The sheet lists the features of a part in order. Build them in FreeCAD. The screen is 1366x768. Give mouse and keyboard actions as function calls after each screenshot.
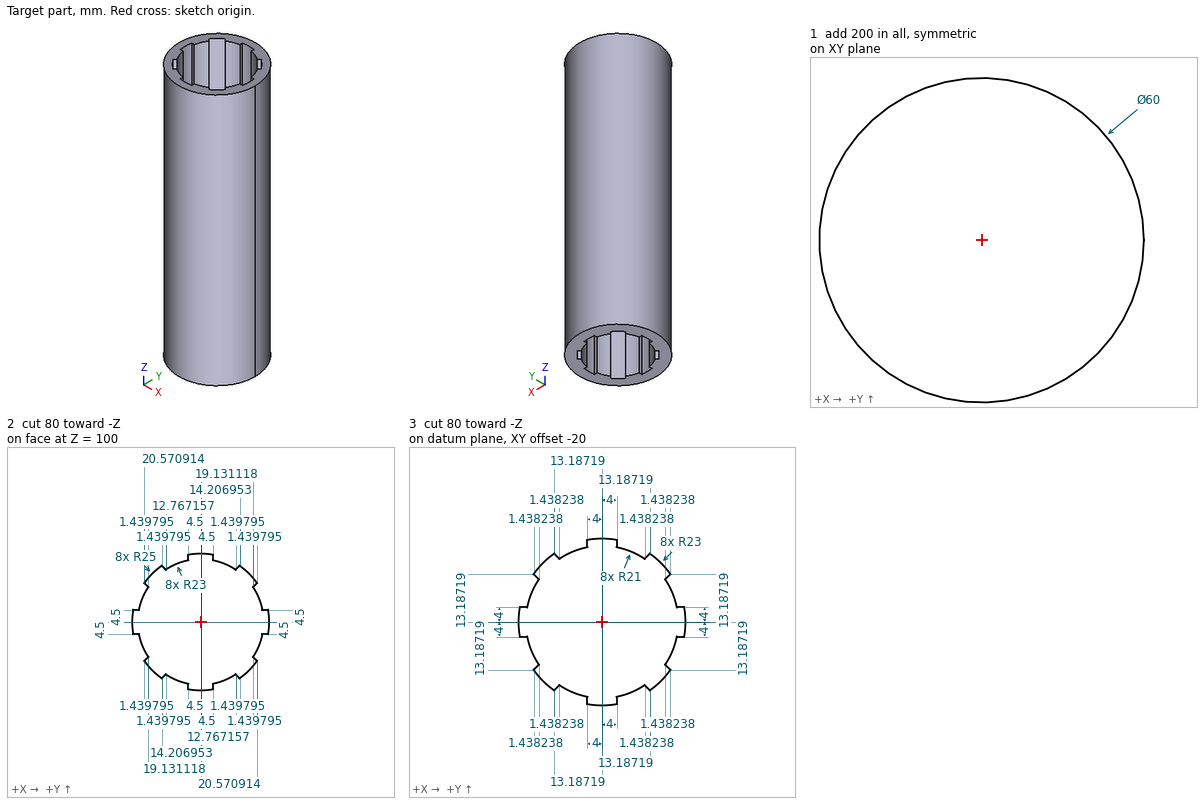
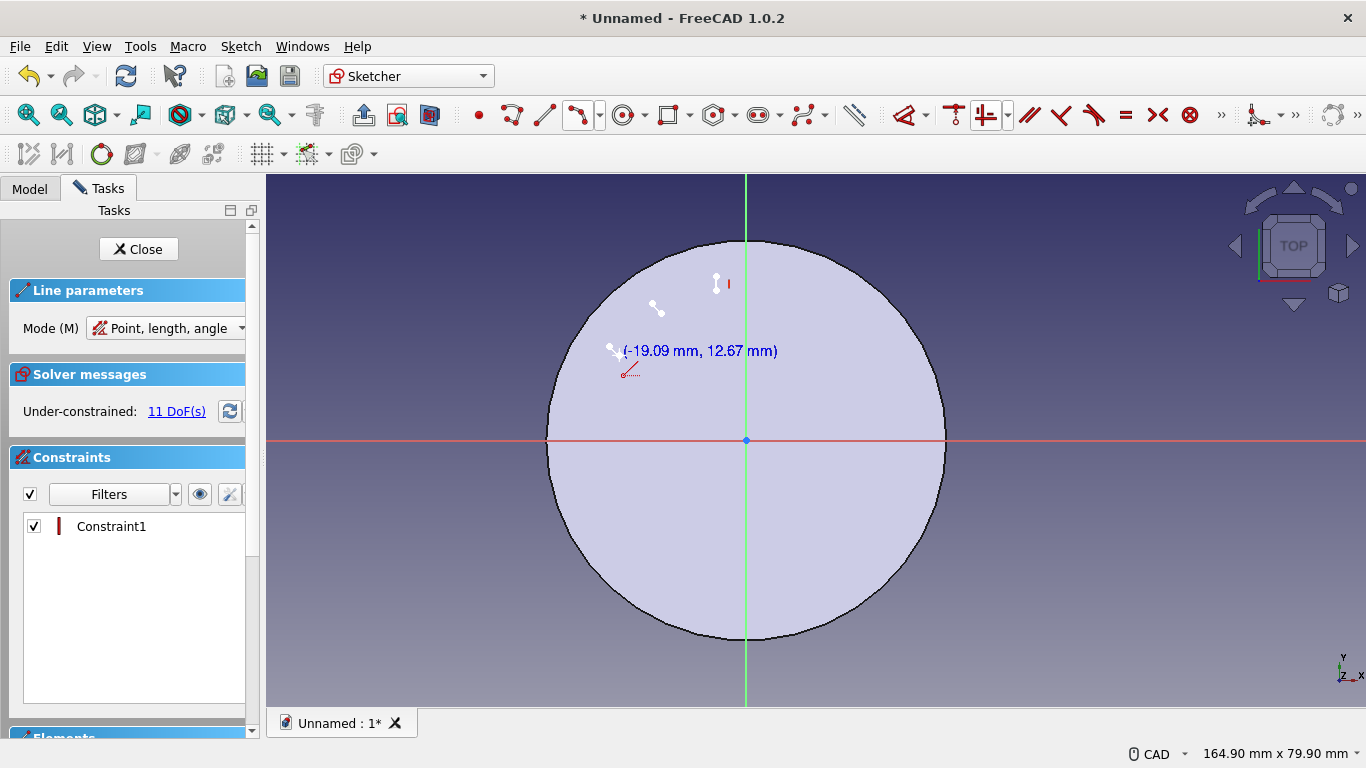
click(596, 410)
click(582, 410)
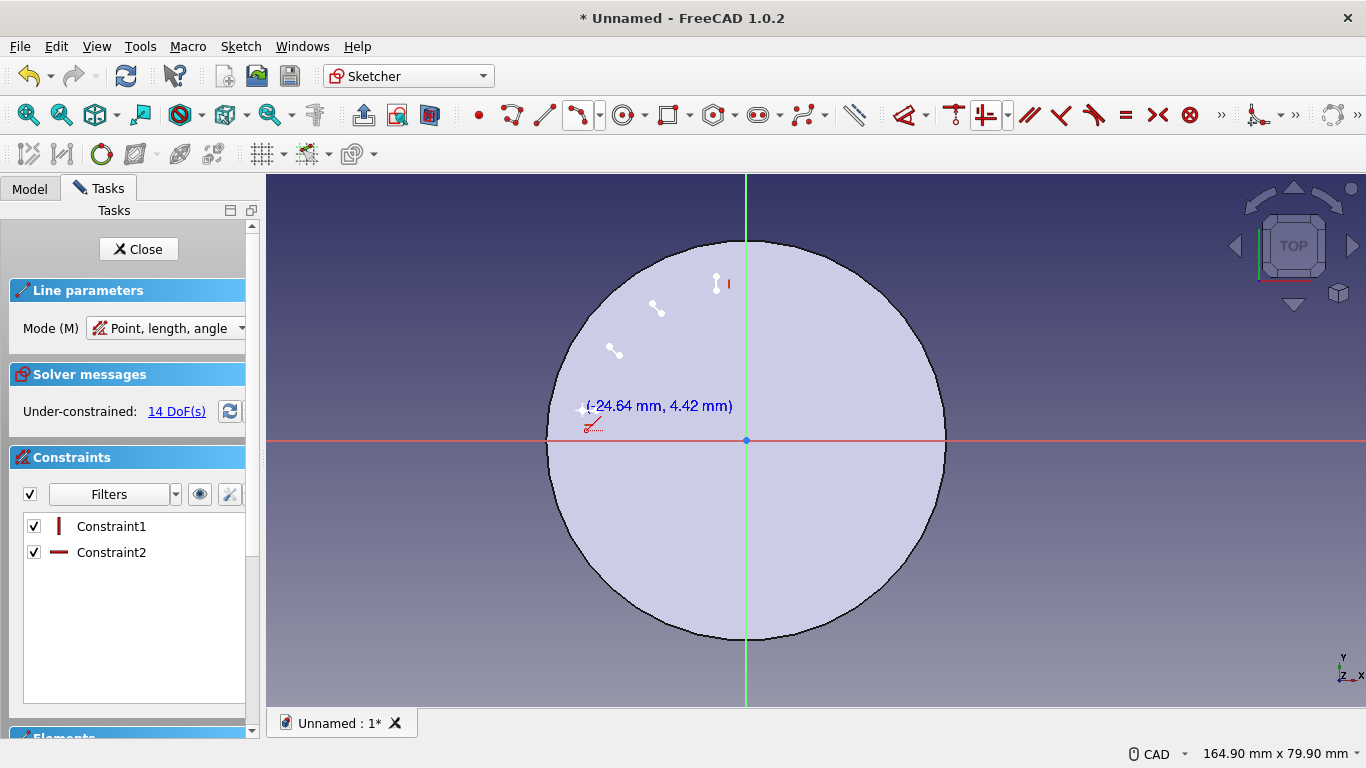
click(582, 471)
click(596, 471)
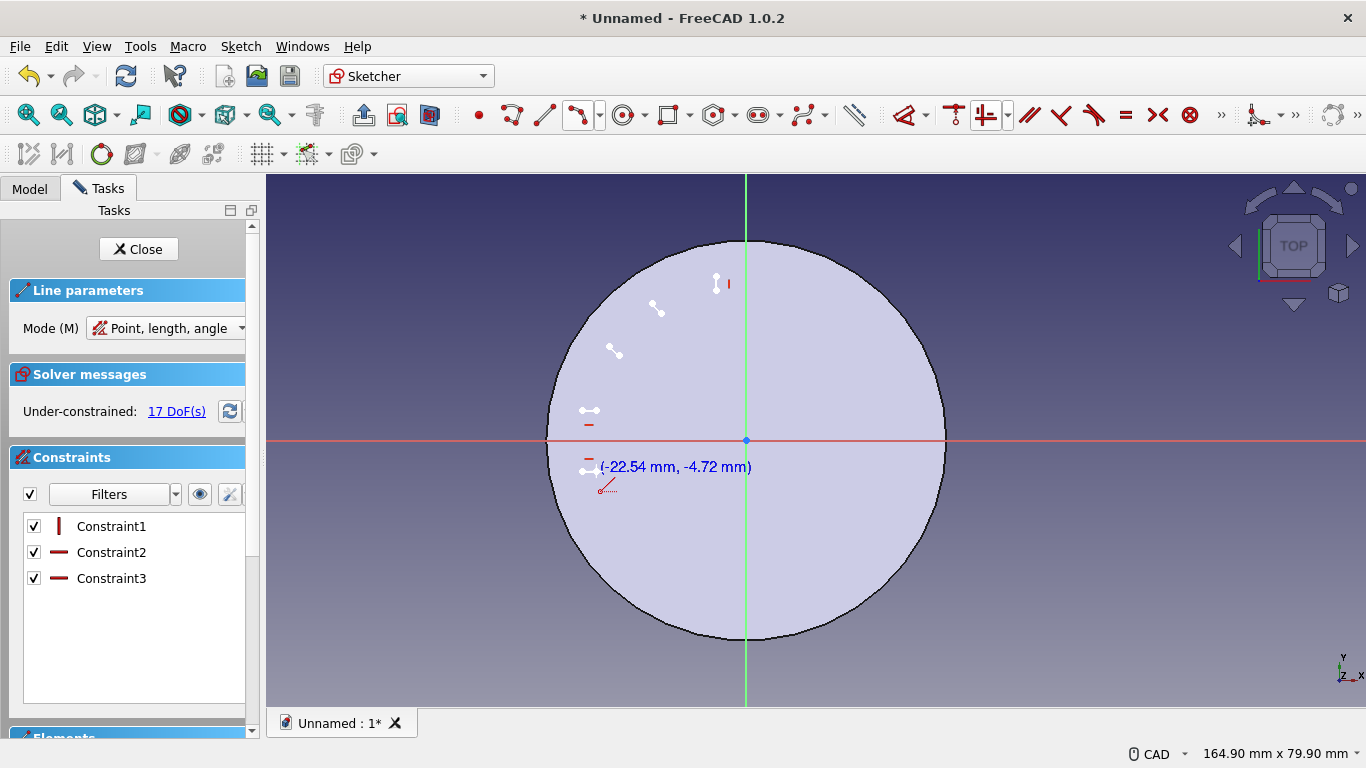
click(619, 526)
click(609, 535)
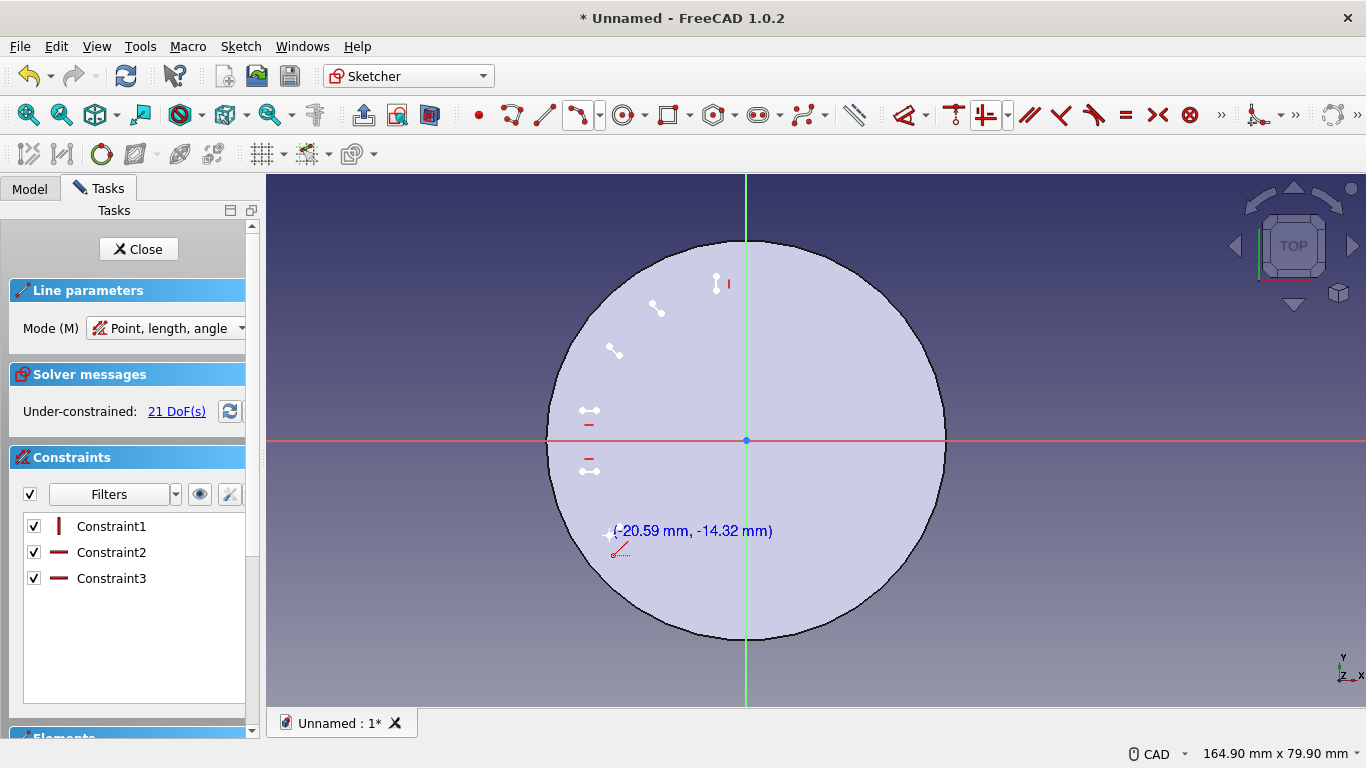
click(652, 578)
click(661, 568)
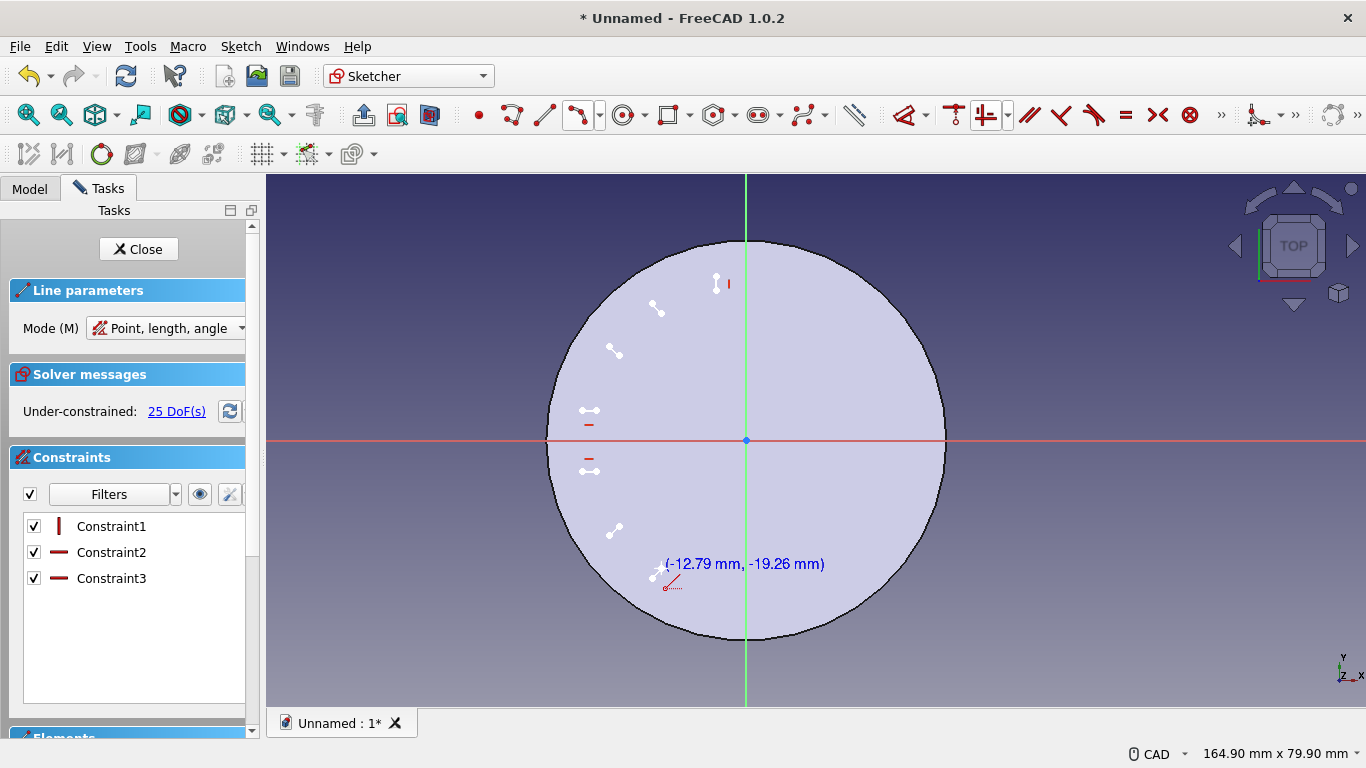
click(716, 591)
click(716, 605)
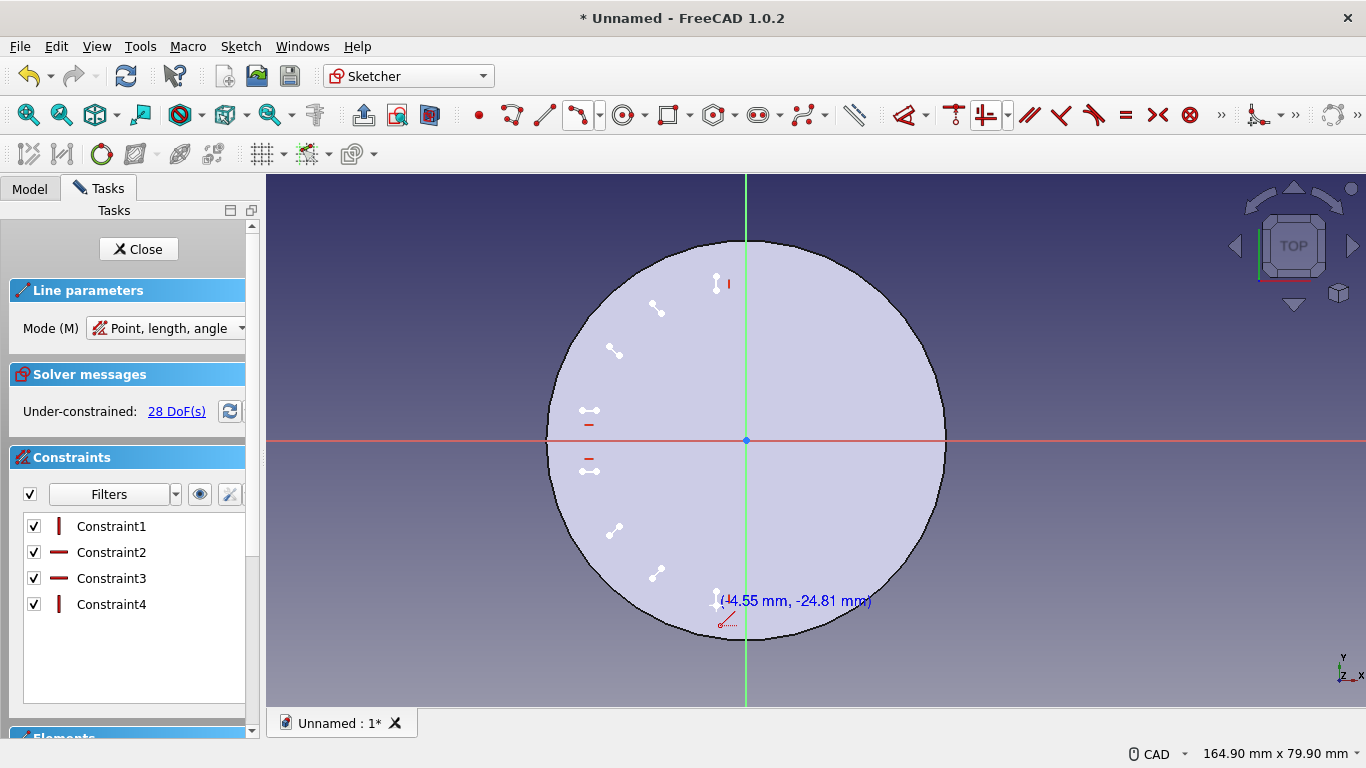
click(776, 605)
click(776, 591)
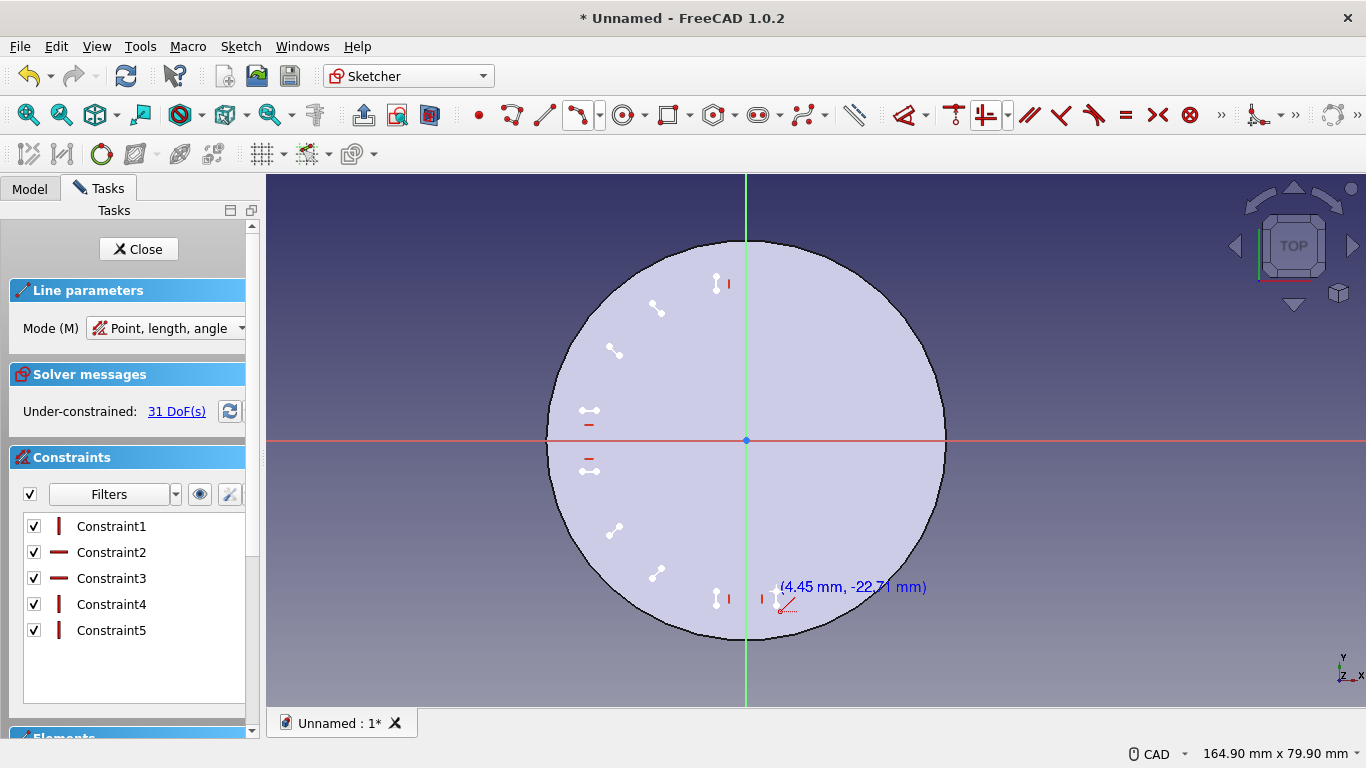
click(832, 568)
click(841, 578)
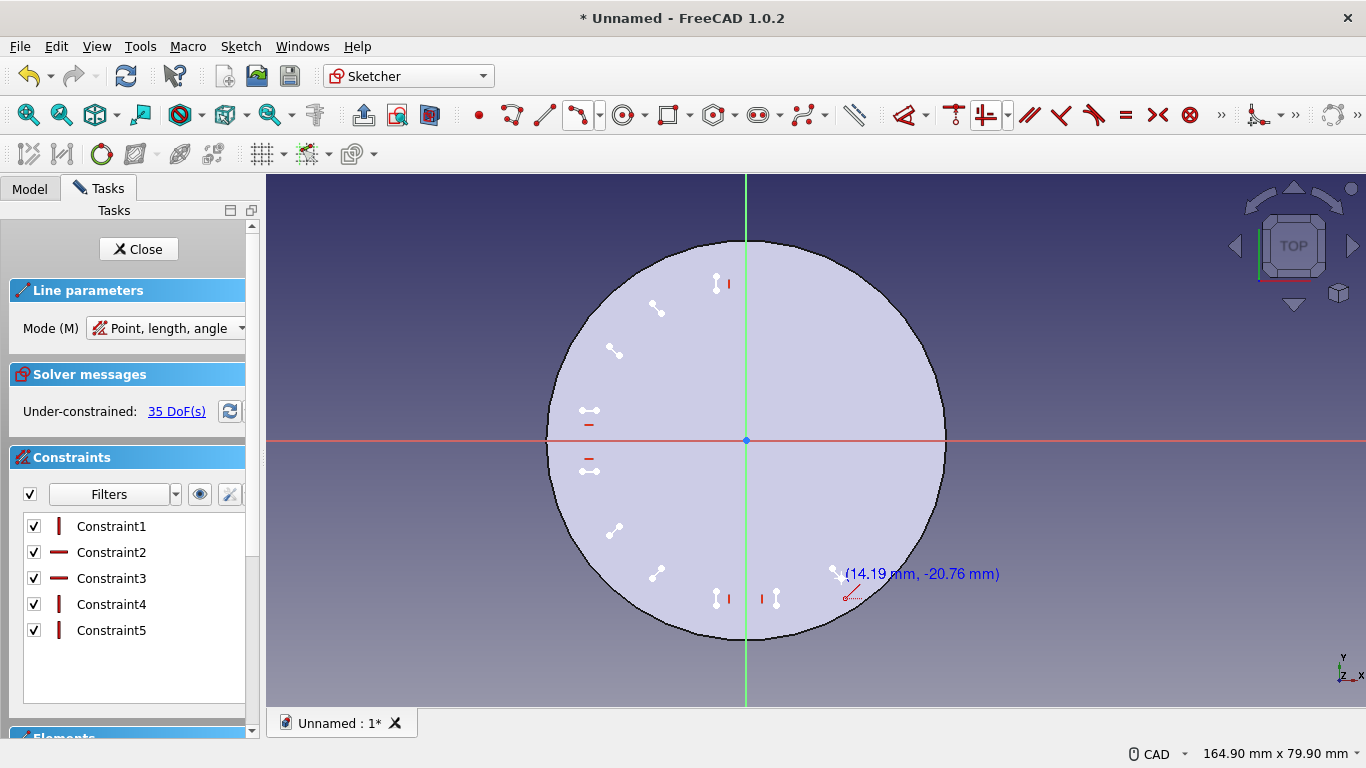
click(884, 535)
click(874, 526)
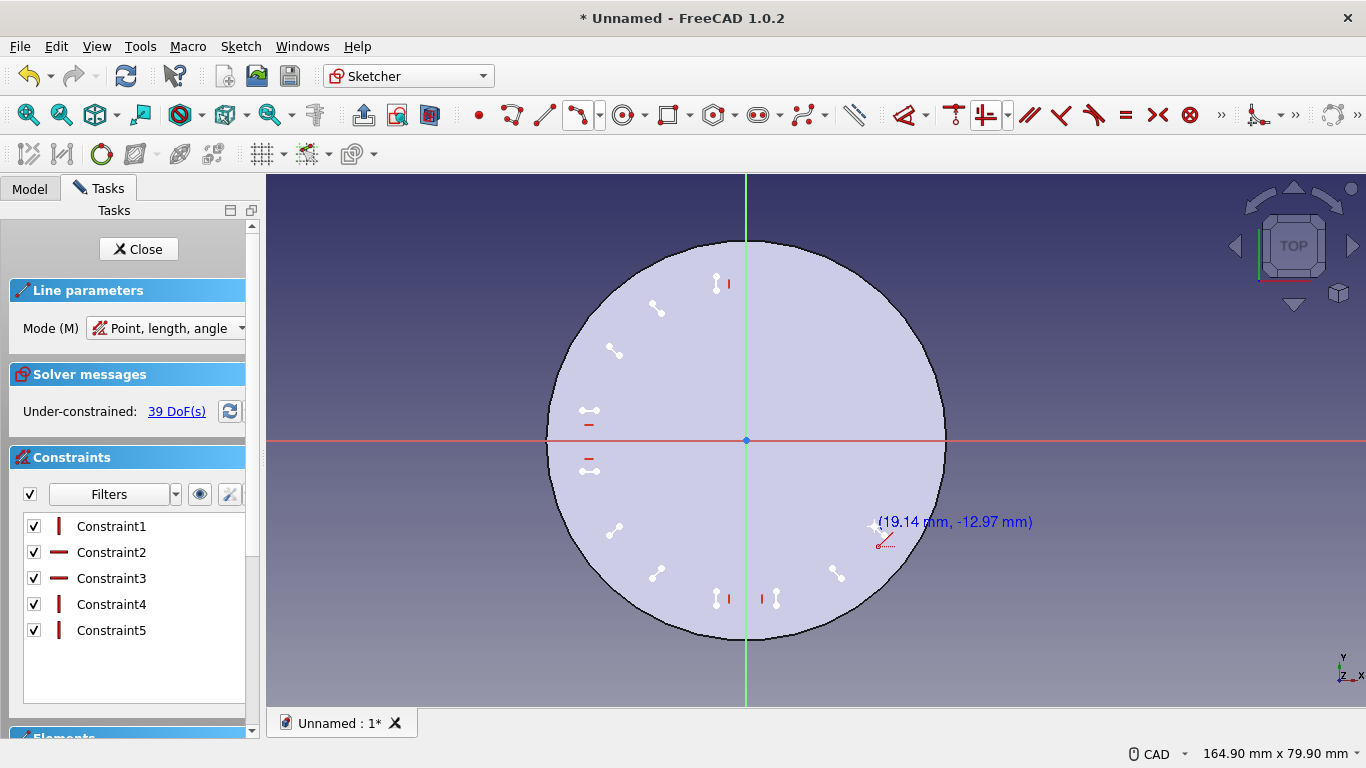
click(897, 471)
click(910, 471)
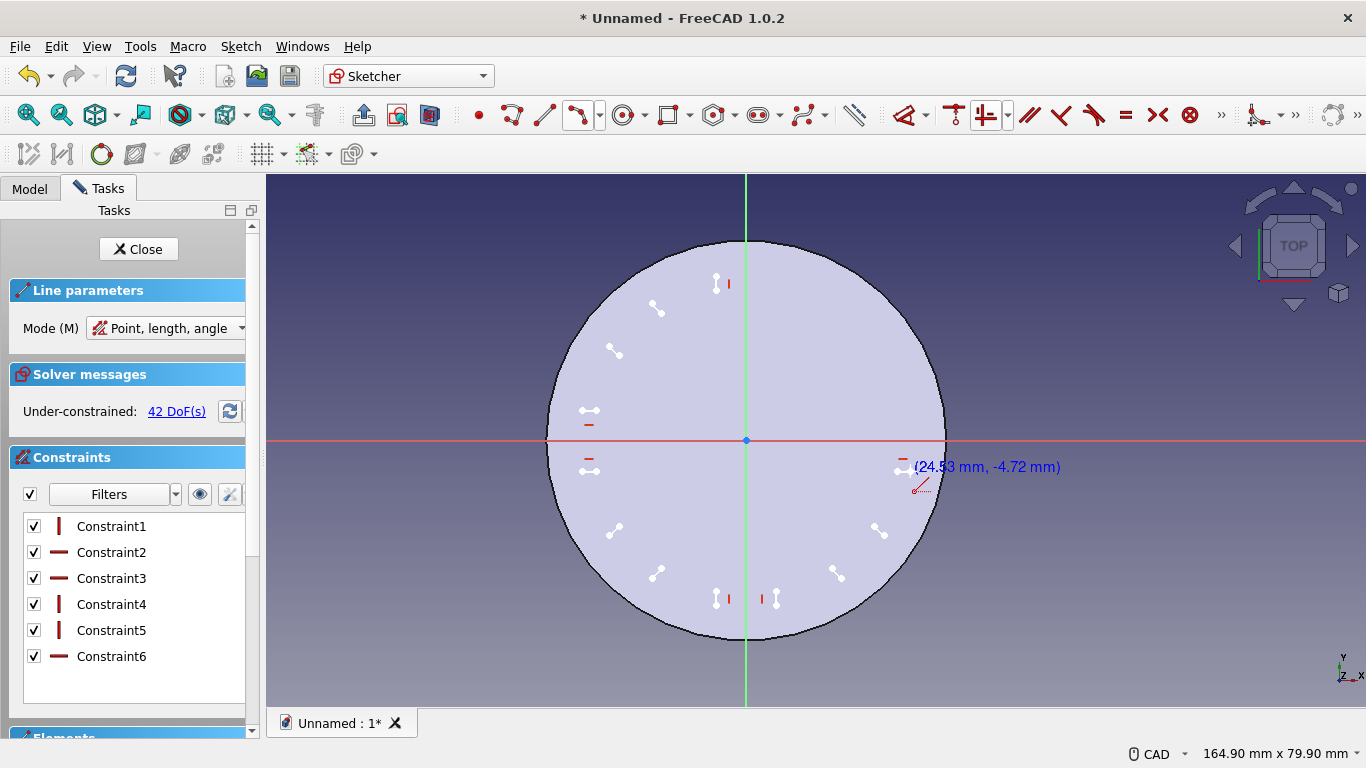
click(910, 410)
click(897, 410)